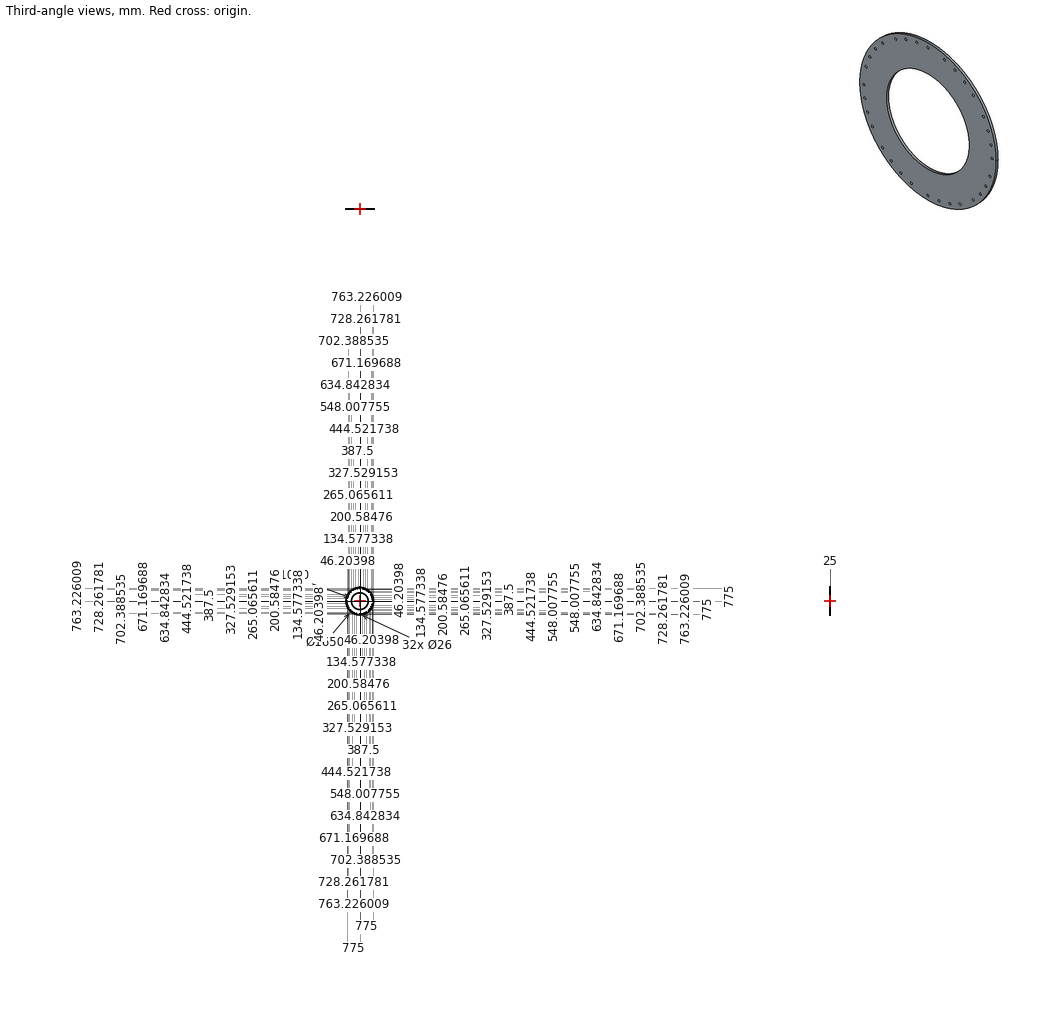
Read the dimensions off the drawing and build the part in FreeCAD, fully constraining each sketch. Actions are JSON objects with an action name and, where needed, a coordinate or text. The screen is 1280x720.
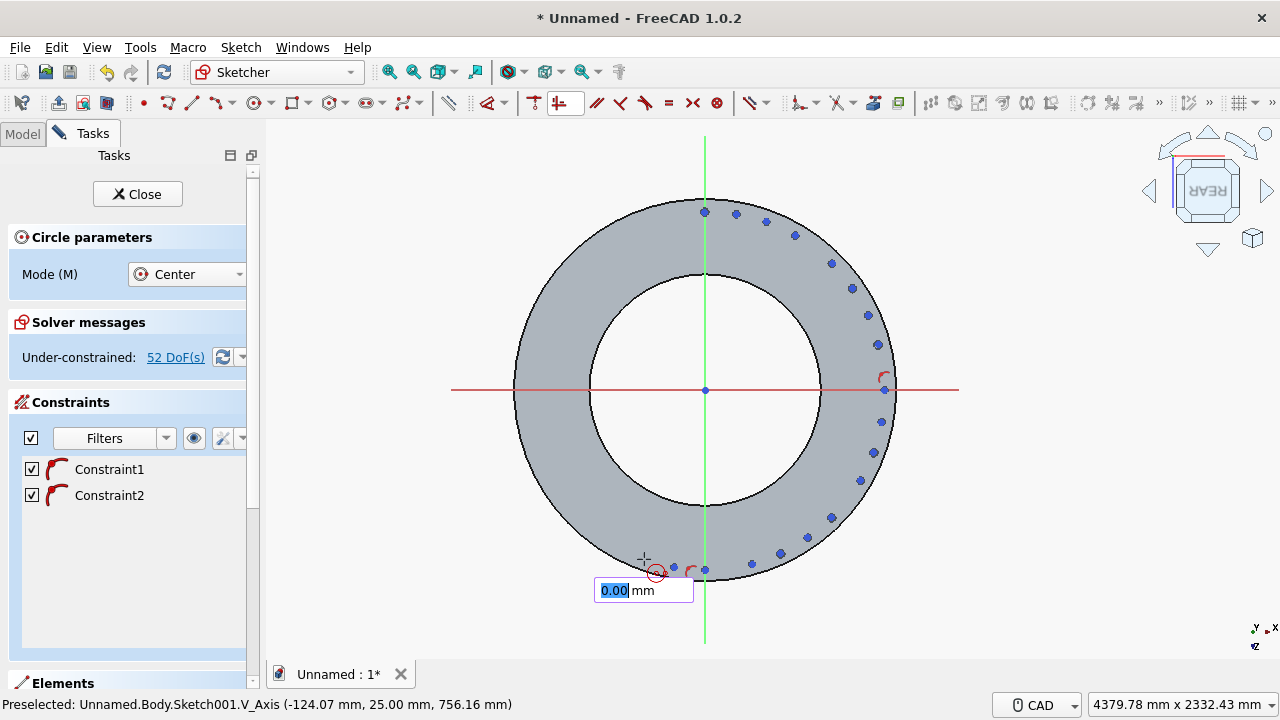
{"action": "scroll", "coordinate": [646, 557], "scroll_direction": "up", "scroll_amount": 9}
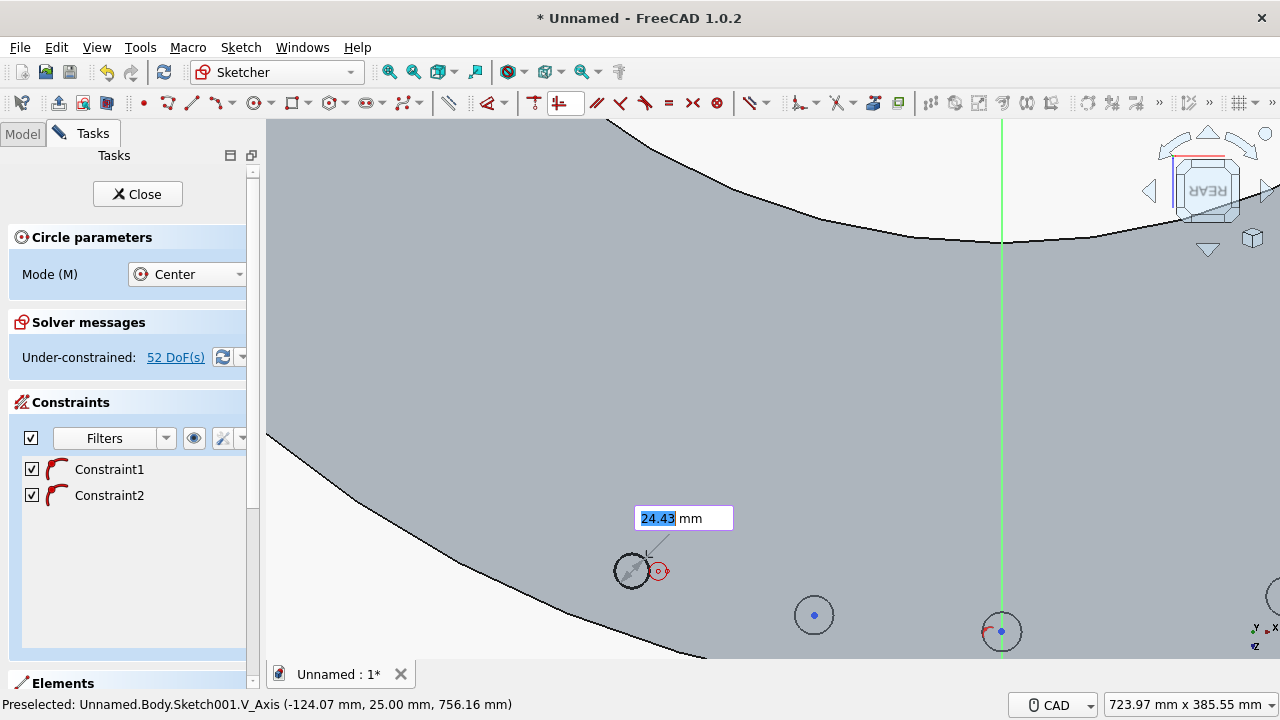
{"action": "left_click", "coordinate": [644, 550]}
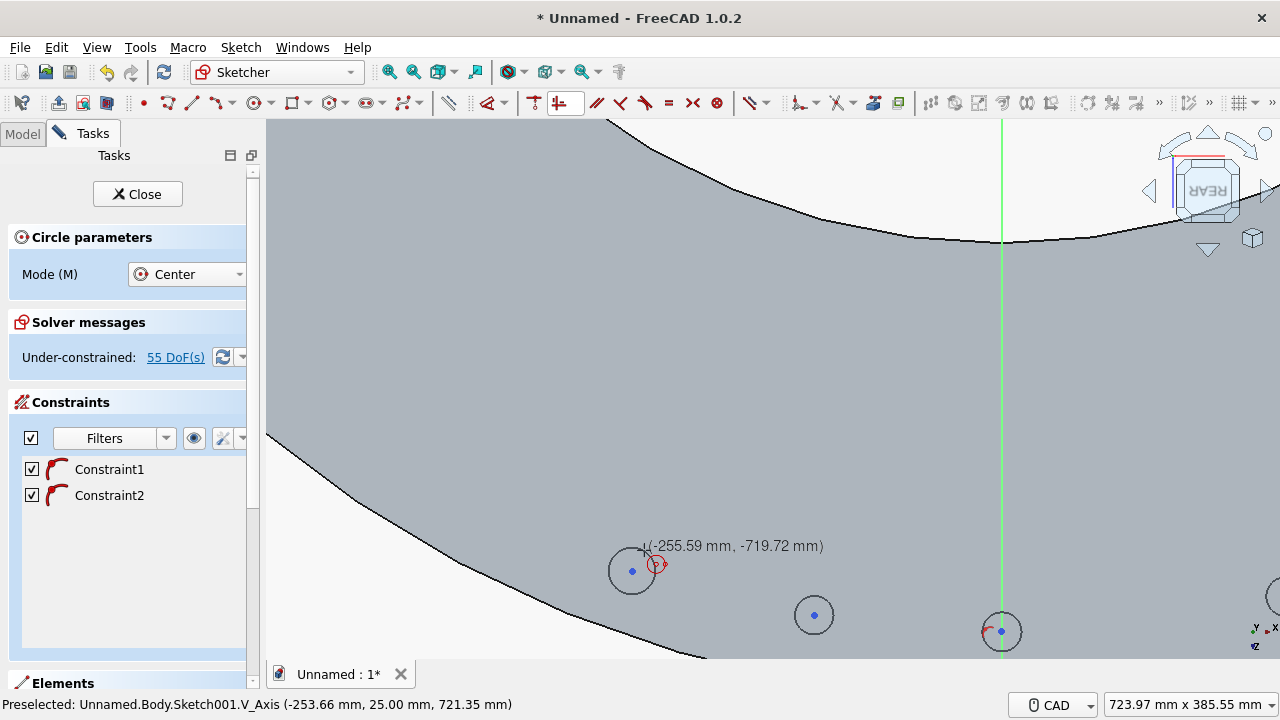
{"action": "scroll", "coordinate": [459, 483], "scroll_direction": "up", "scroll_amount": 2}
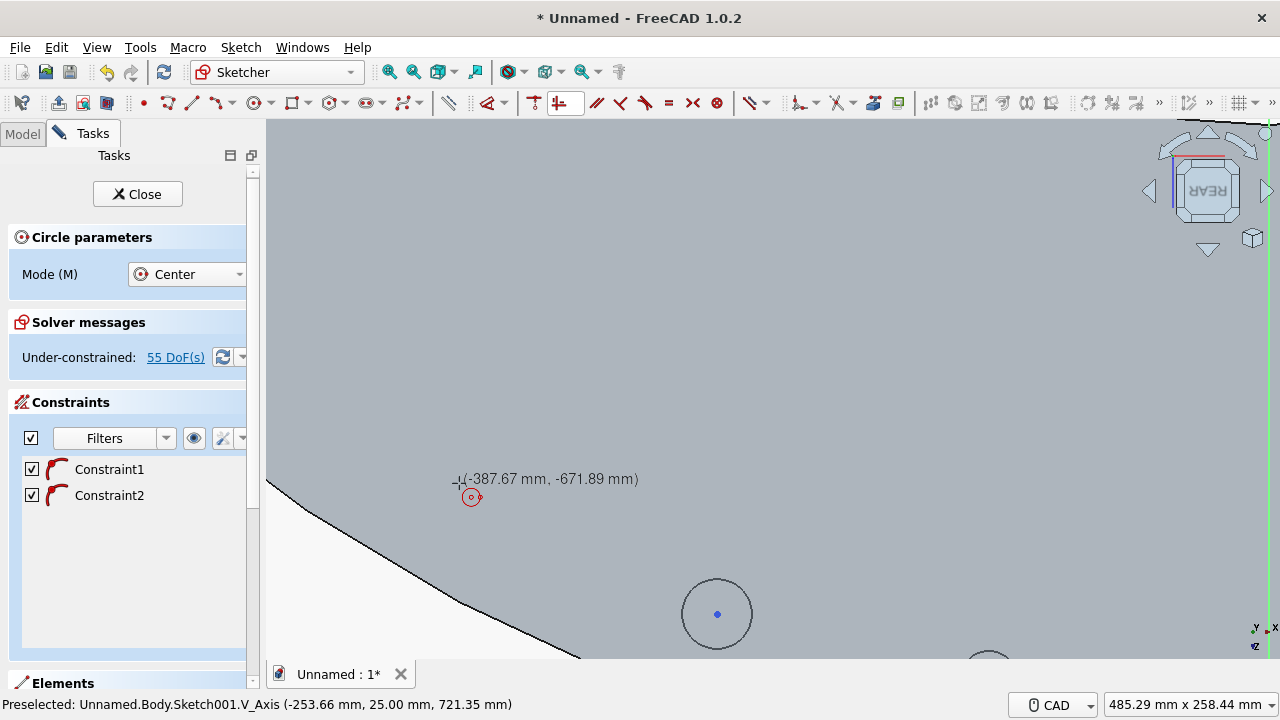
{"action": "scroll", "coordinate": [634, 552], "scroll_direction": "down", "scroll_amount": 11}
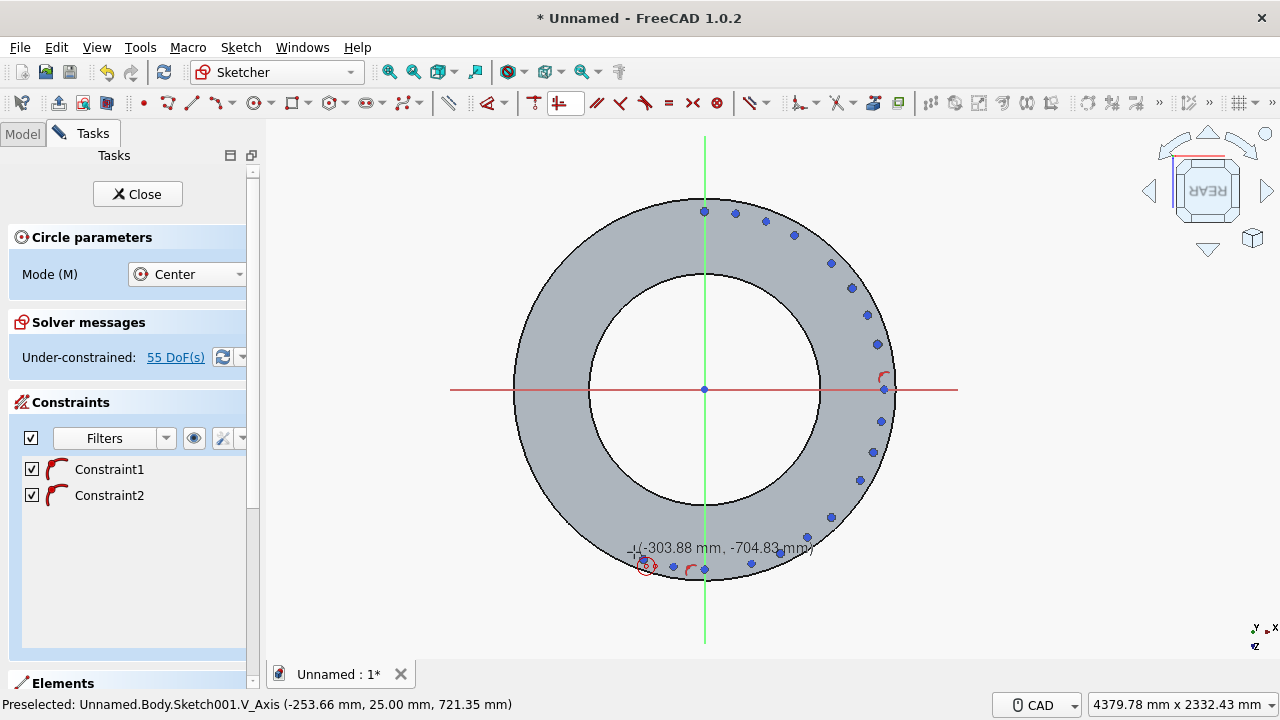
{"action": "left_click", "coordinate": [615, 545]}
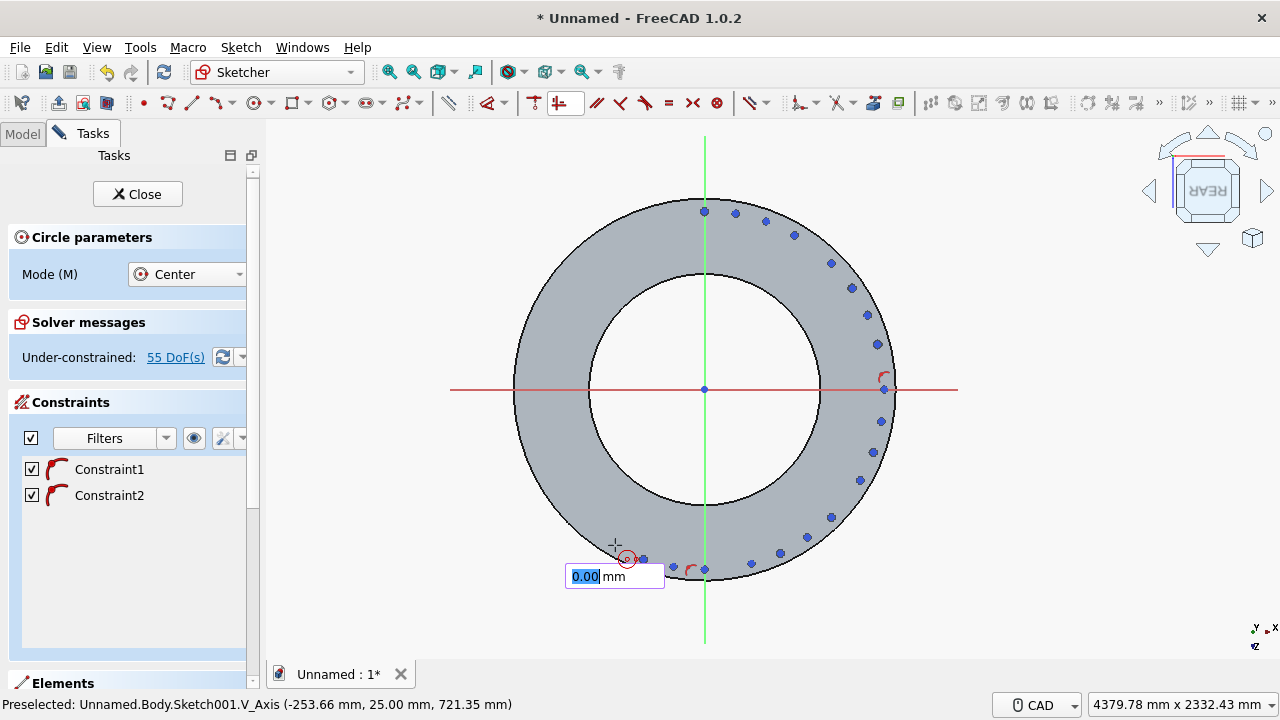
{"action": "scroll", "coordinate": [617, 543], "scroll_direction": "up", "scroll_amount": 9}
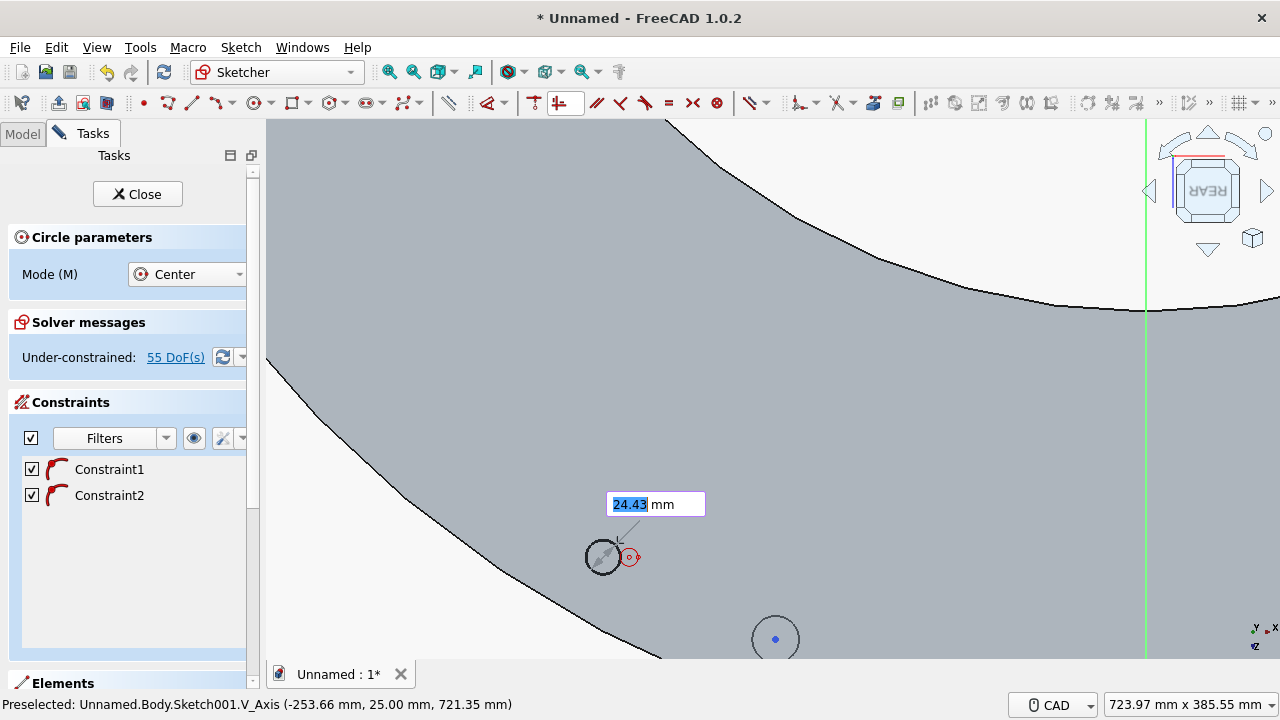
{"action": "left_click", "coordinate": [616, 538]}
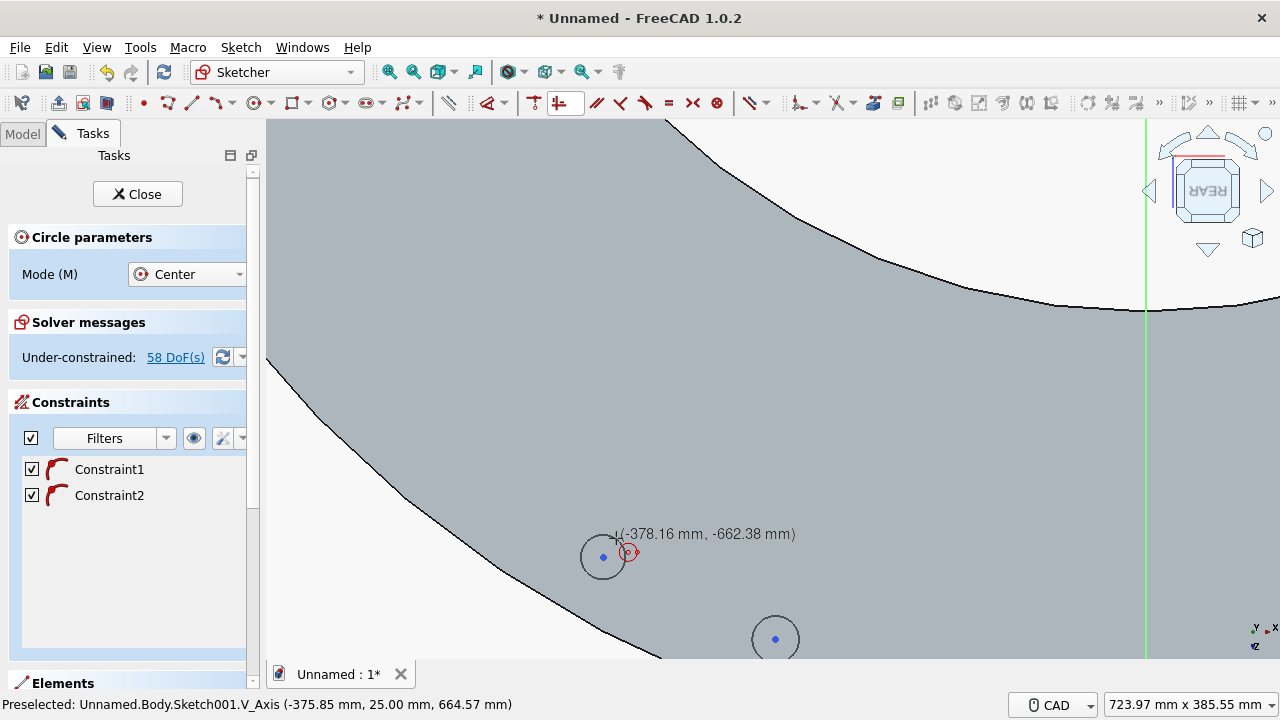
{"action": "scroll", "coordinate": [378, 379], "scroll_direction": "up", "scroll_amount": 2}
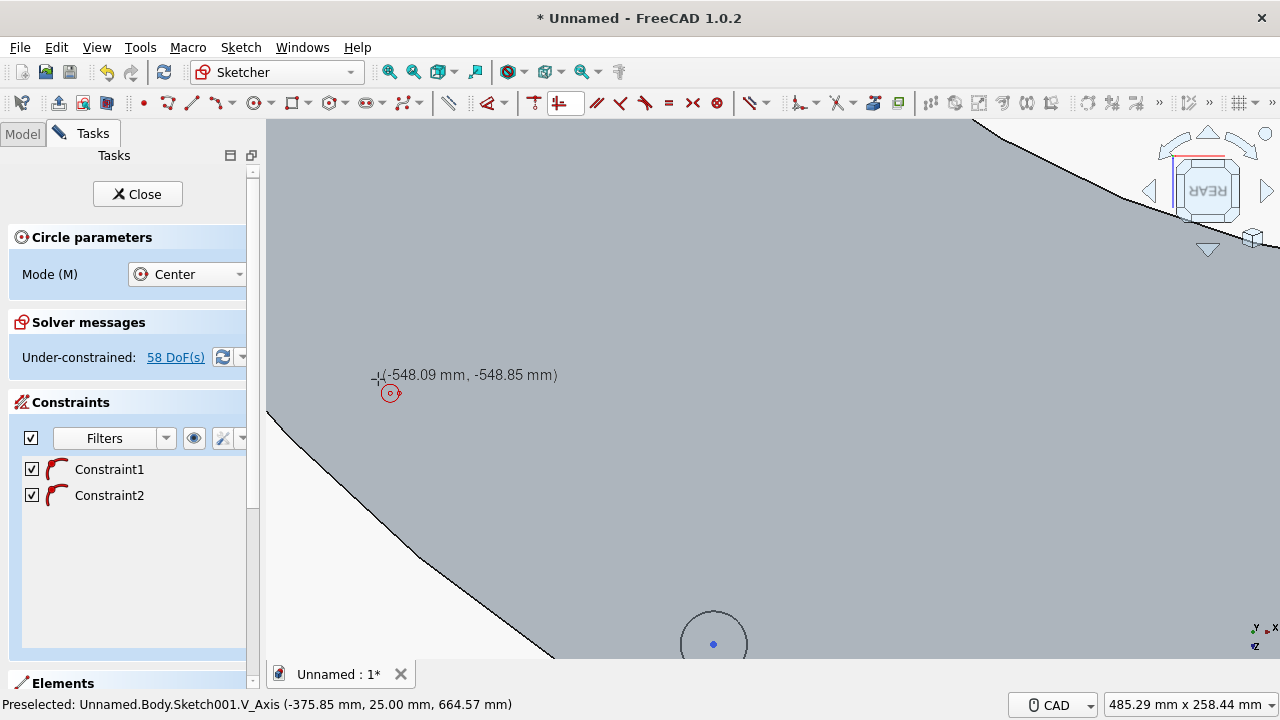
{"action": "scroll", "coordinate": [602, 533], "scroll_direction": "down", "scroll_amount": 11}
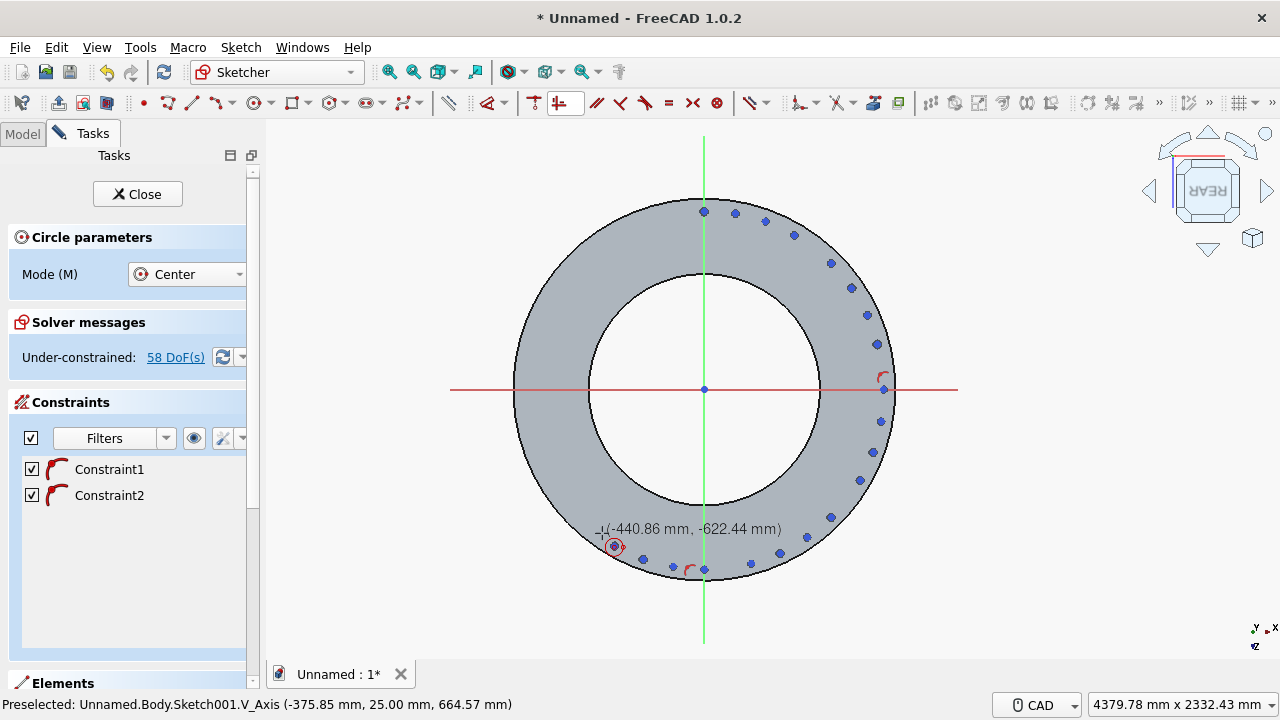
{"action": "left_click", "coordinate": [577, 517]}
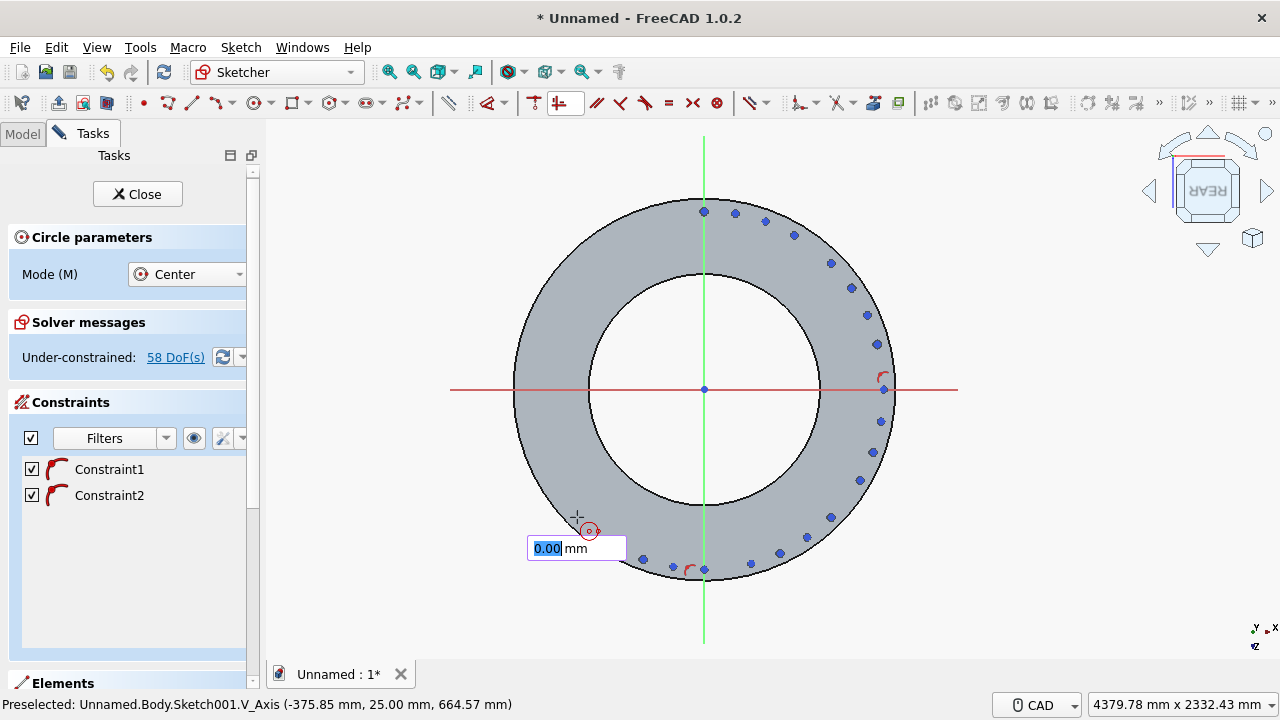
{"action": "scroll", "coordinate": [580, 514], "scroll_direction": "up", "scroll_amount": 9}